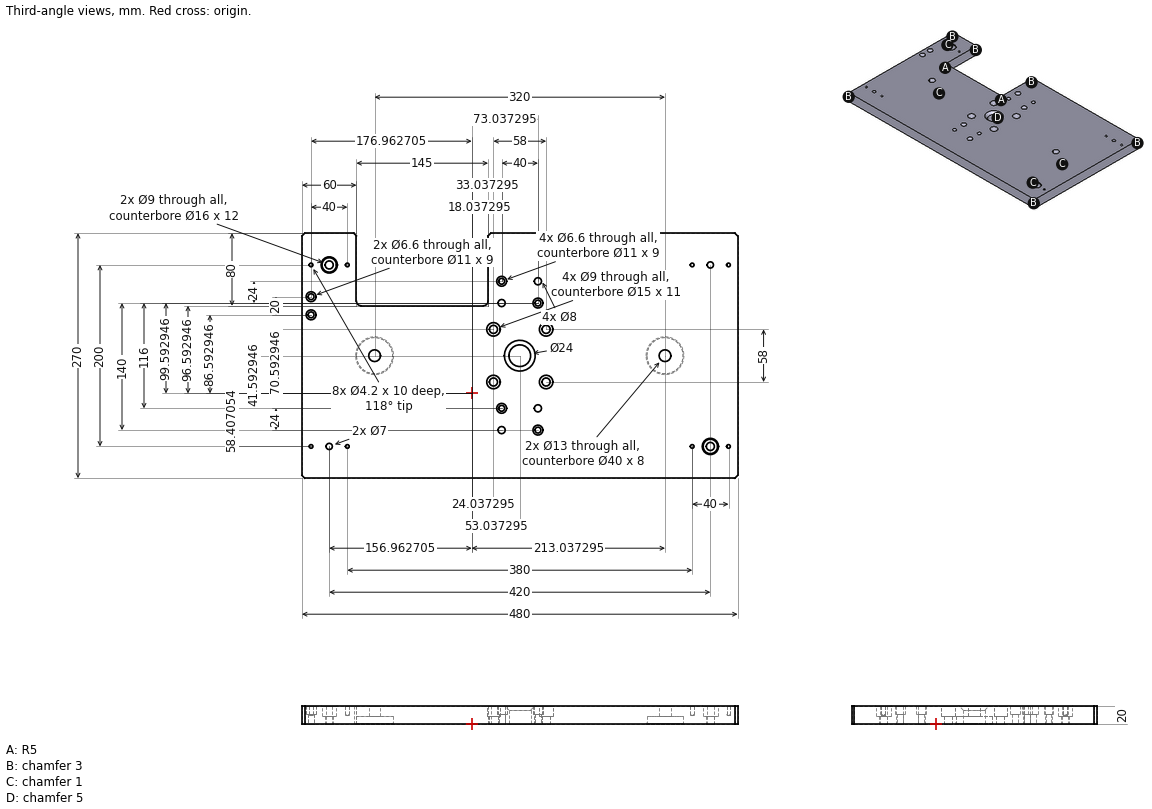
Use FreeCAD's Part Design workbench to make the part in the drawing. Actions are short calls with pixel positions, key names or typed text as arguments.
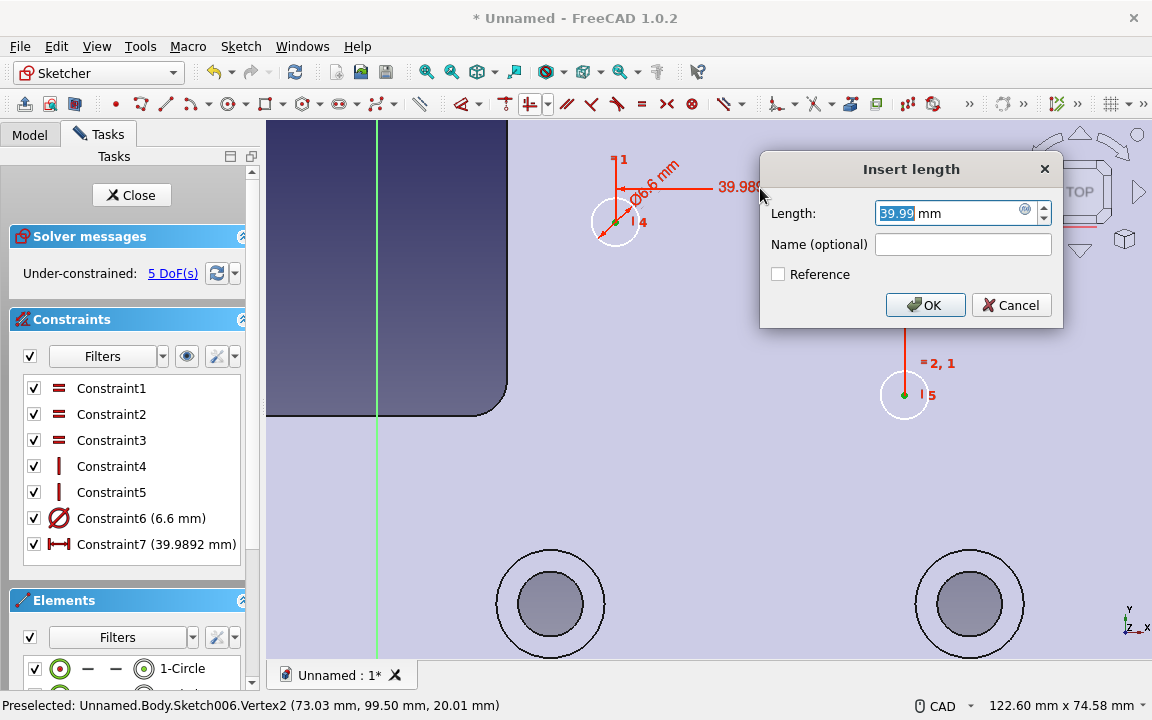
text(40)
key(Return)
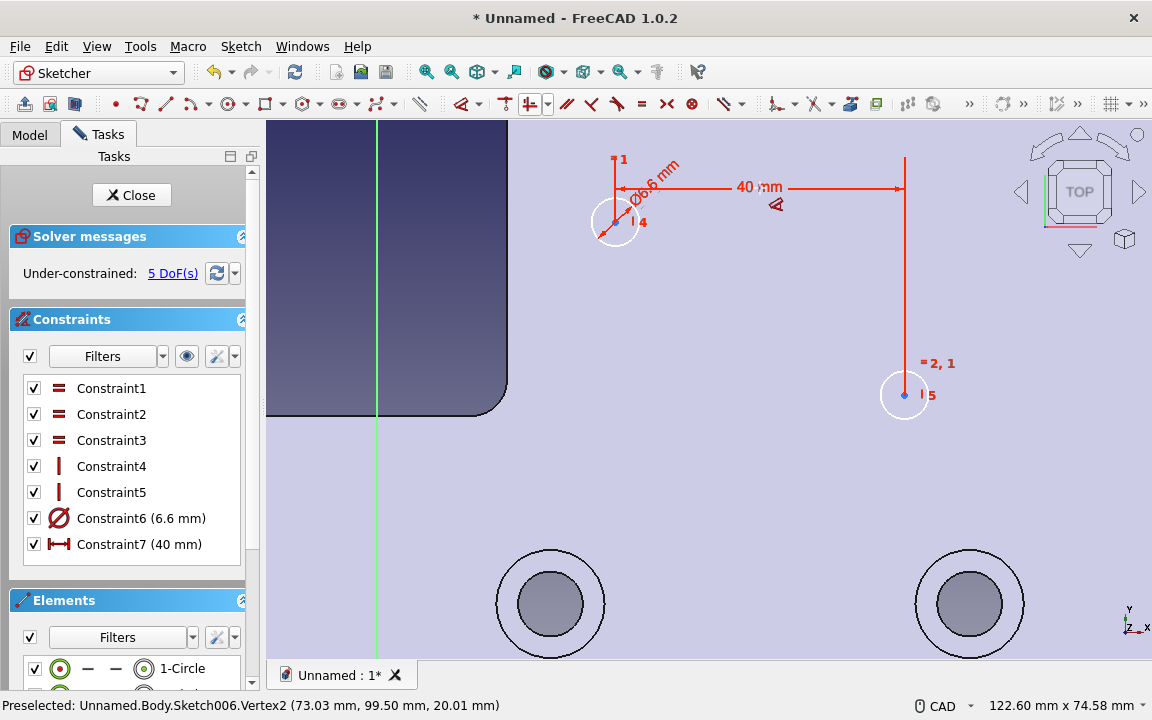
click(615, 222)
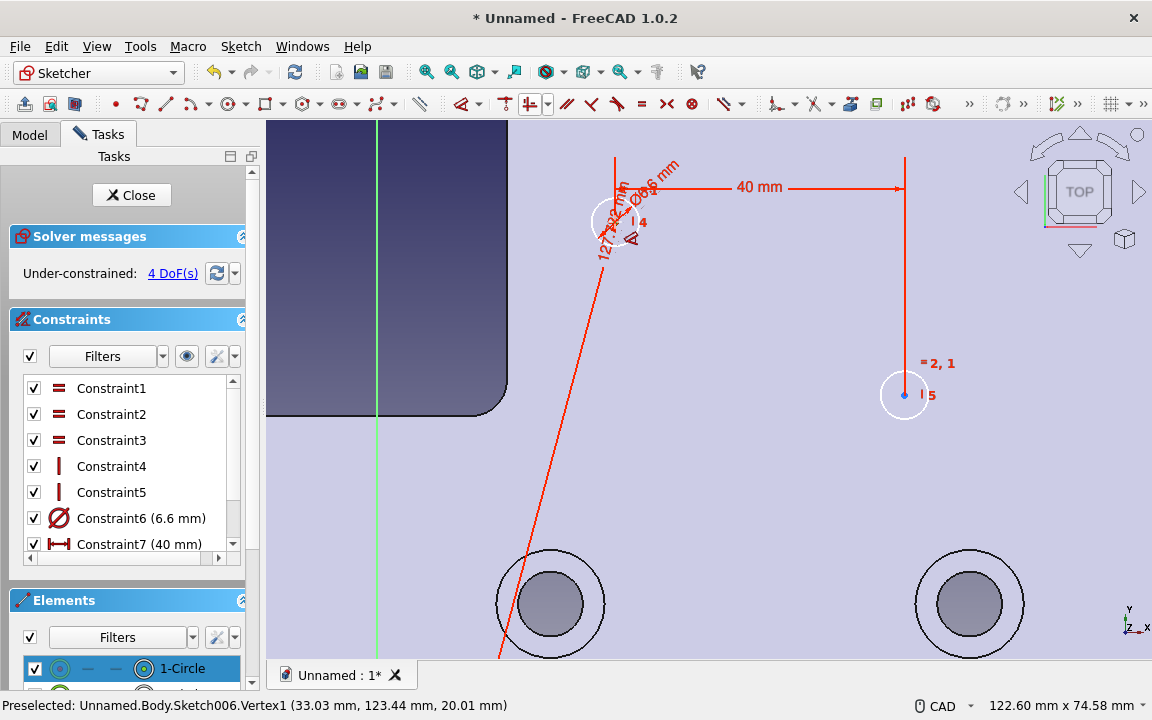
click(905, 395)
click(939, 309)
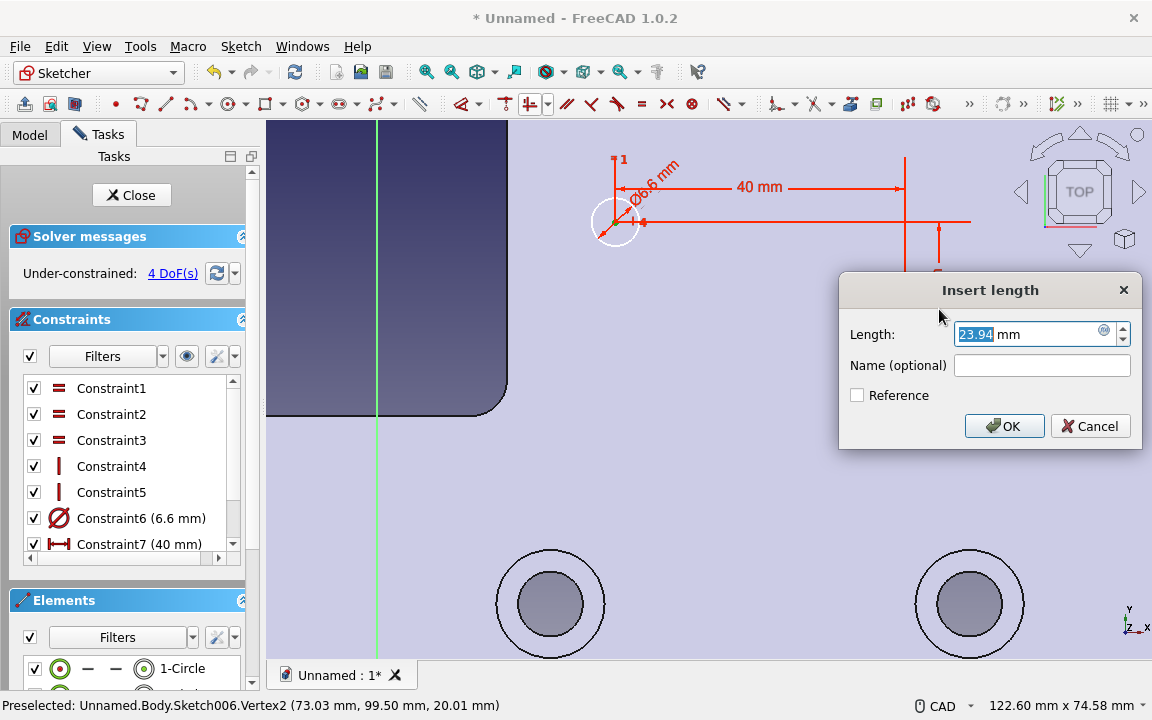
text(24)
key(Return)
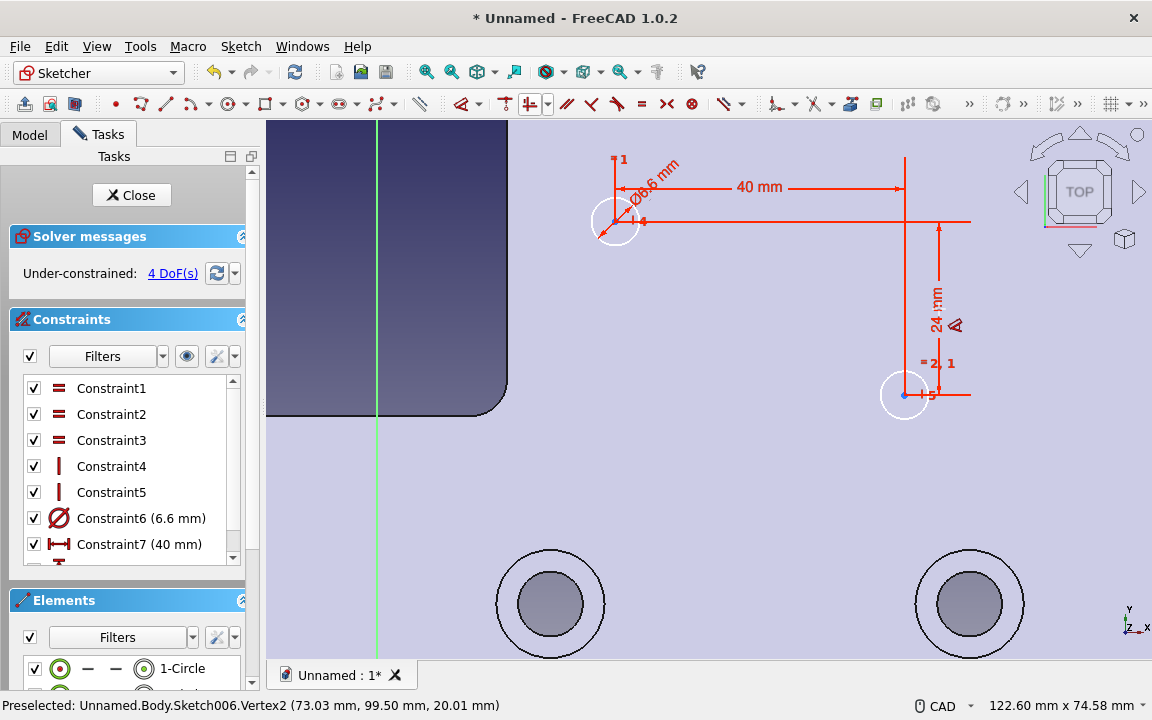
scroll(635, 207, down, 6)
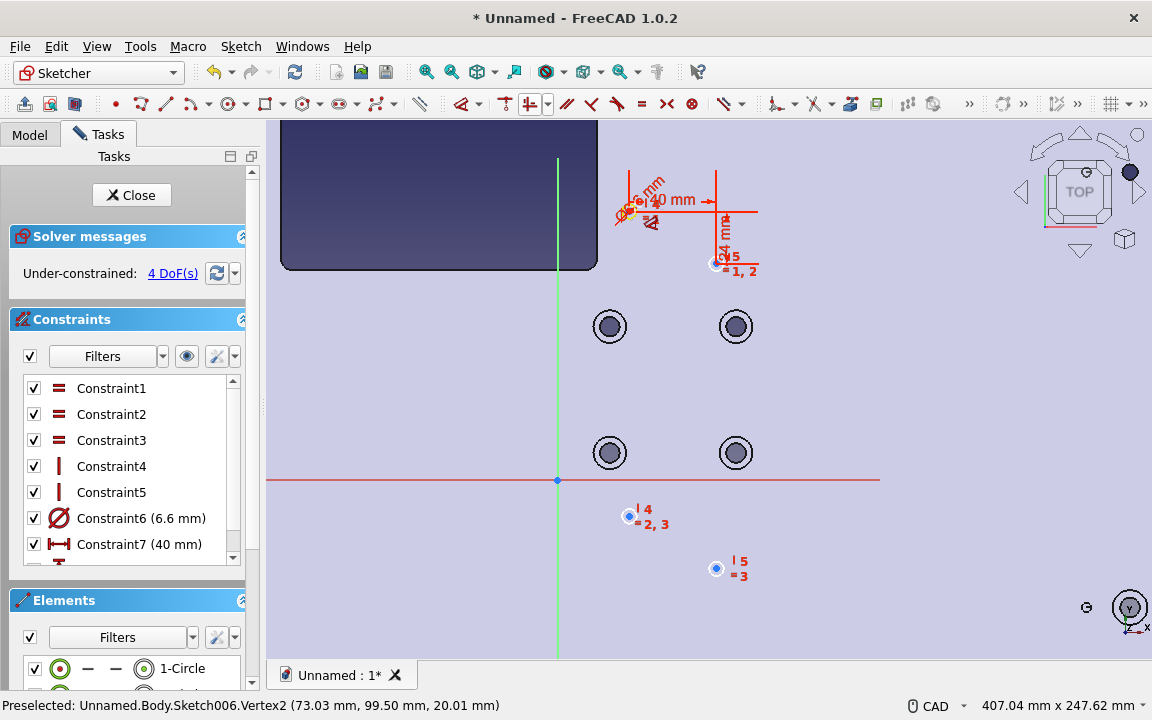
click(629, 516)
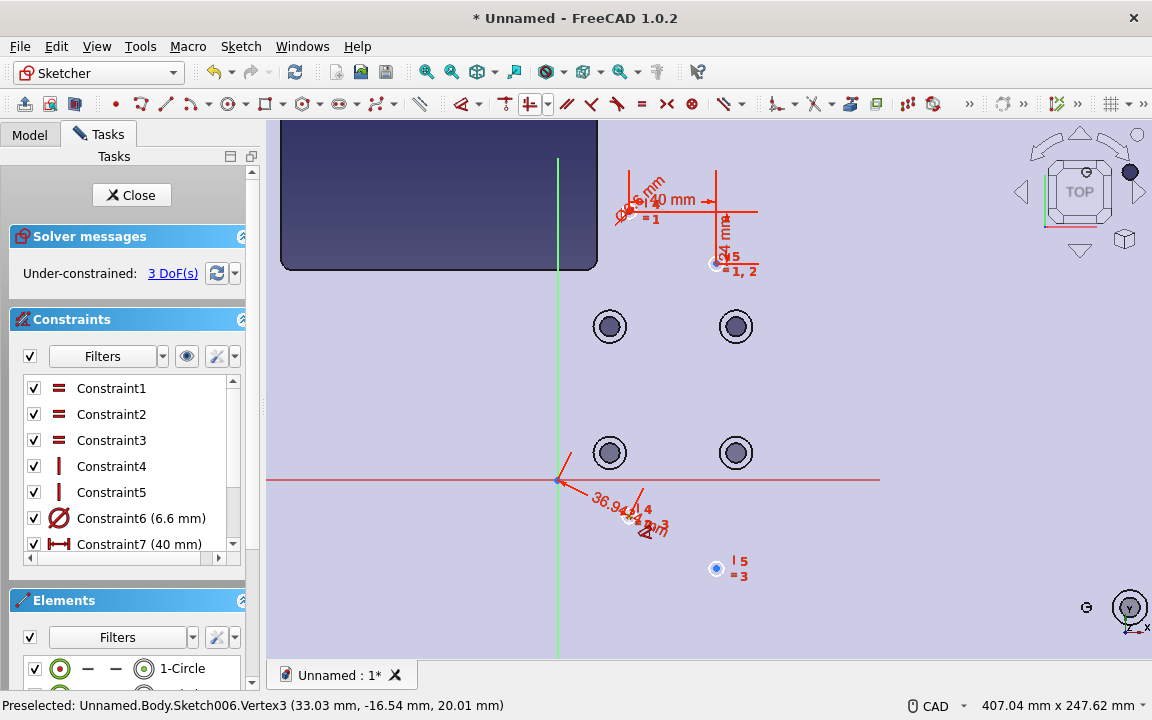
click(716, 569)
click(750, 543)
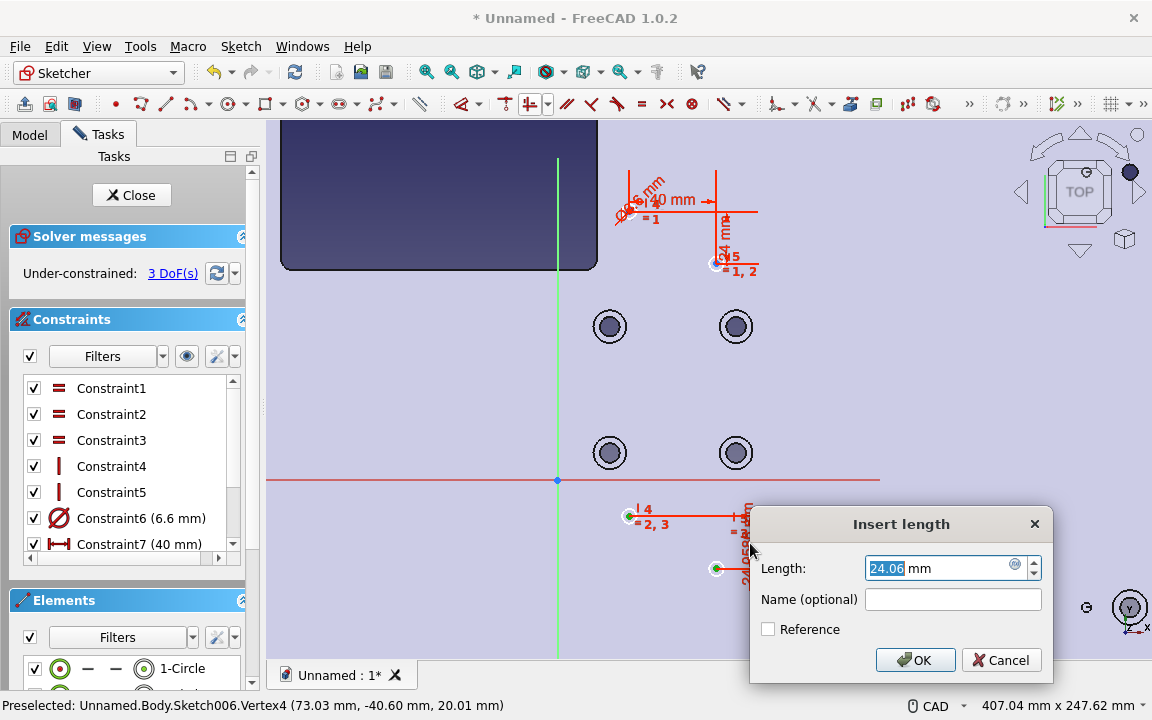
text(24)
key(Return)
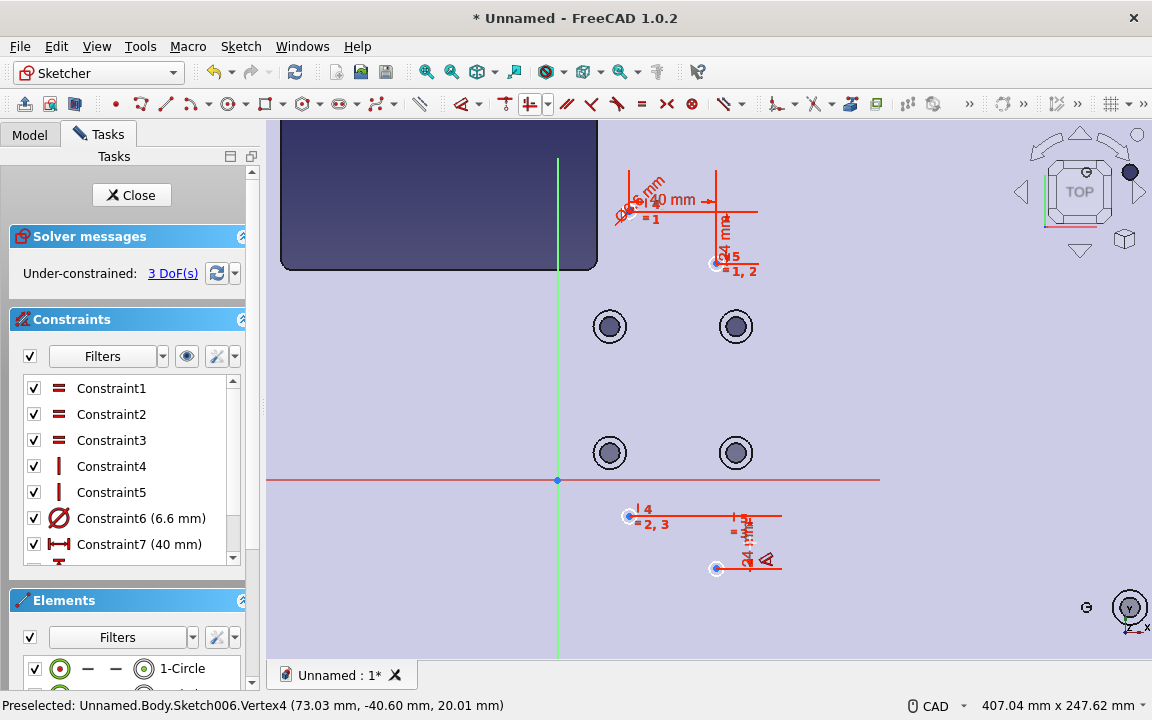
click(716, 264)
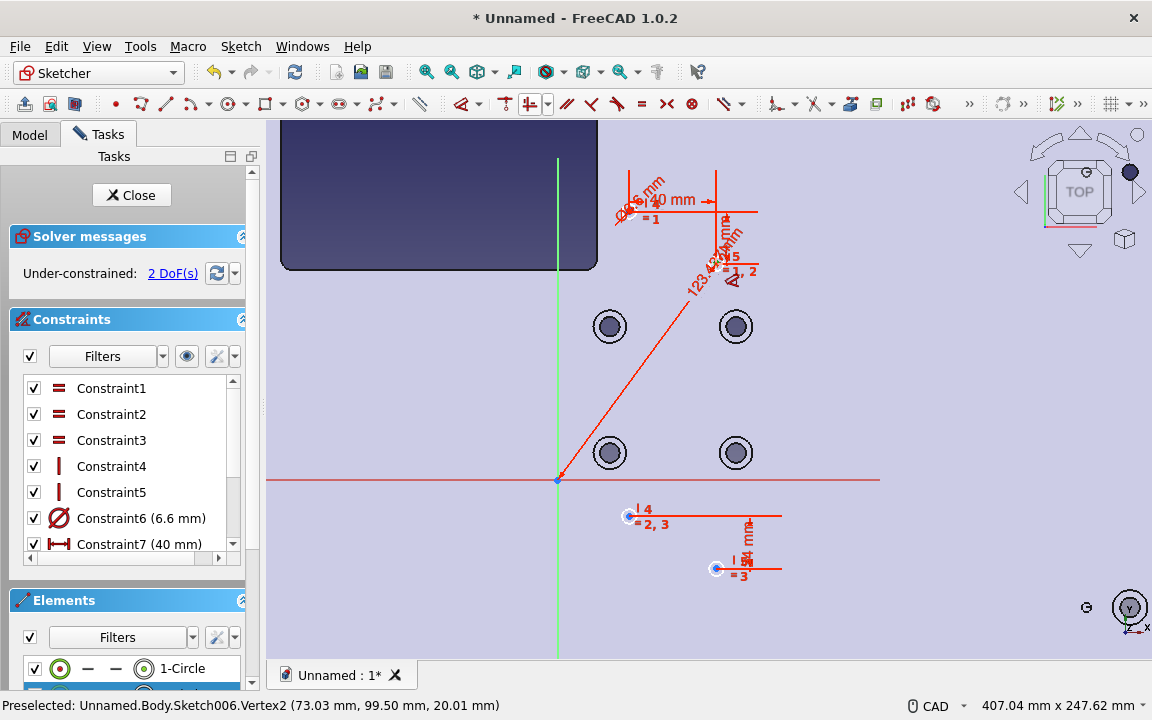
click(629, 516)
click(750, 390)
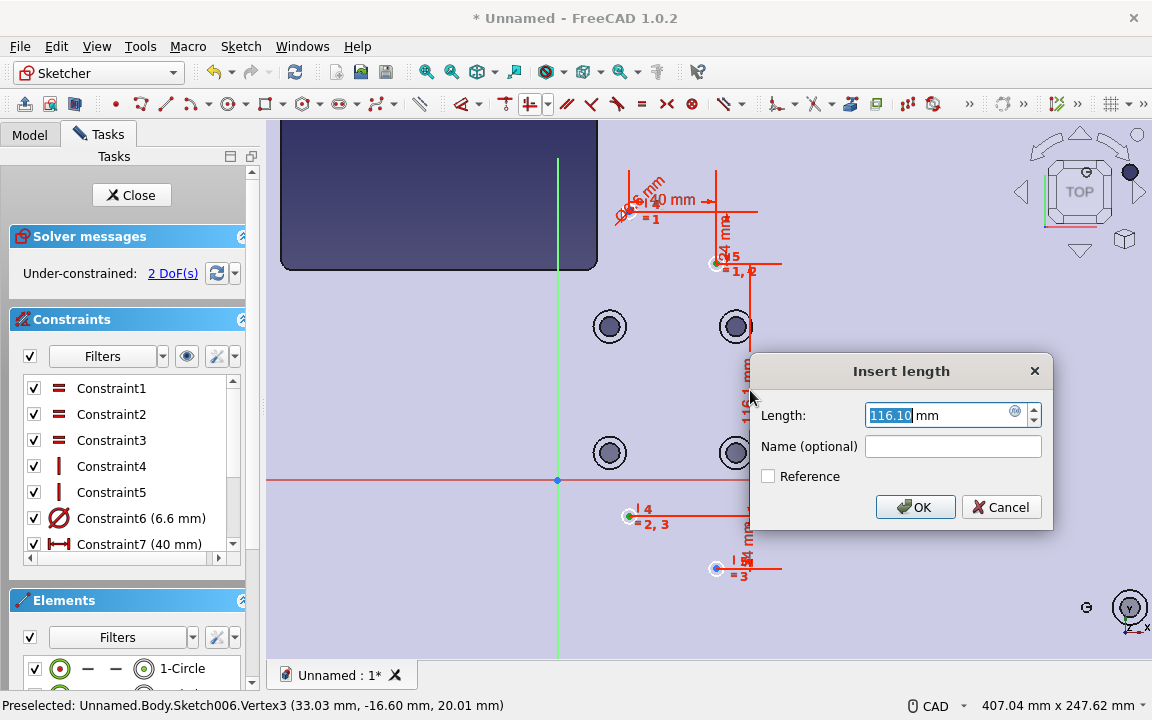
text(116)
key(Return)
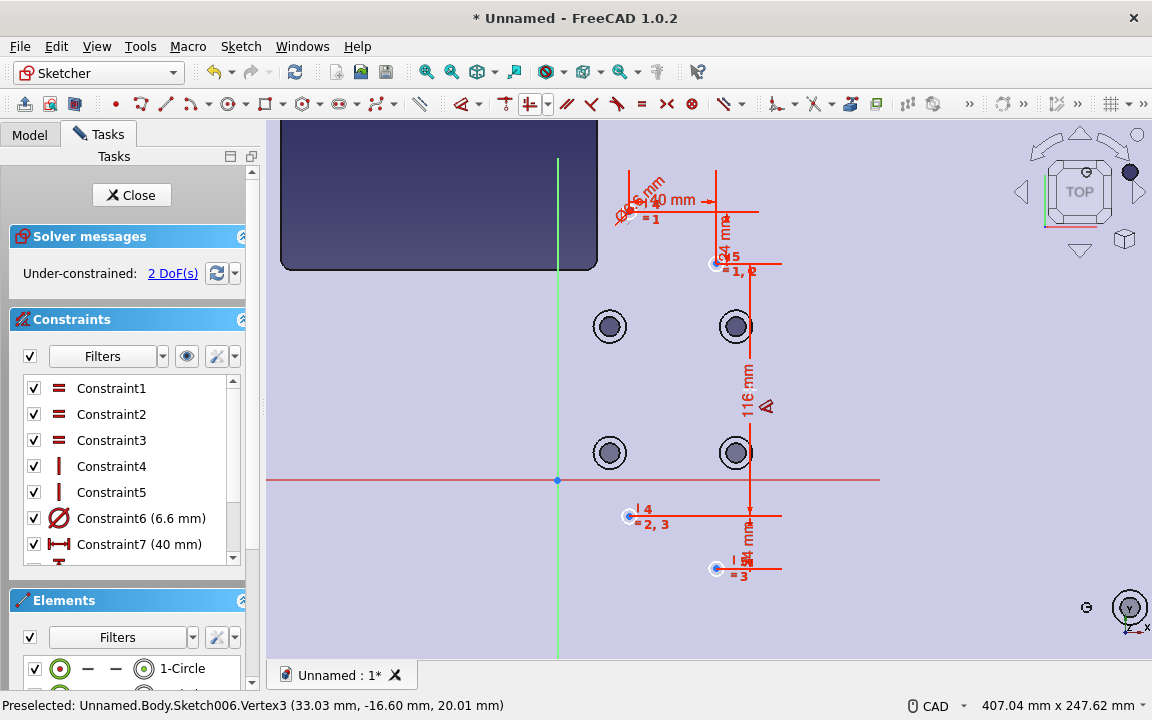
click(629, 212)
click(593, 178)